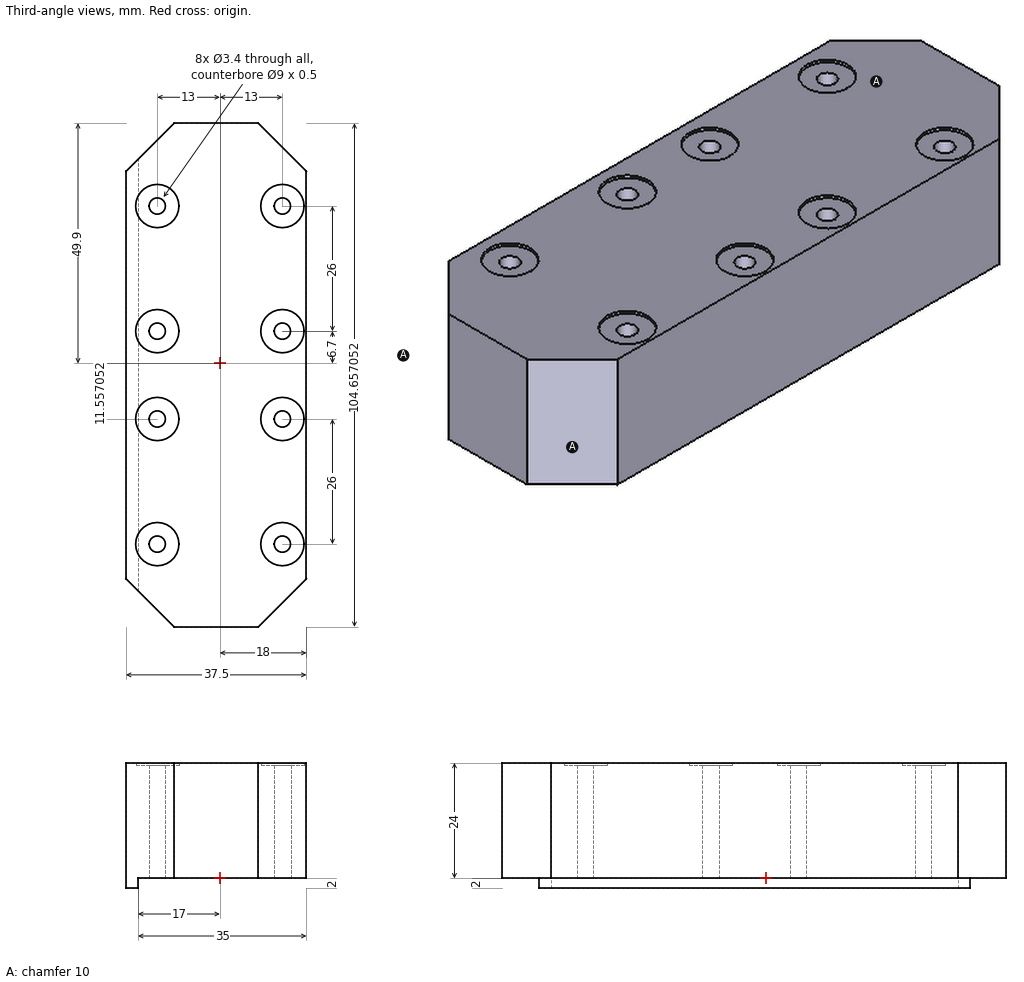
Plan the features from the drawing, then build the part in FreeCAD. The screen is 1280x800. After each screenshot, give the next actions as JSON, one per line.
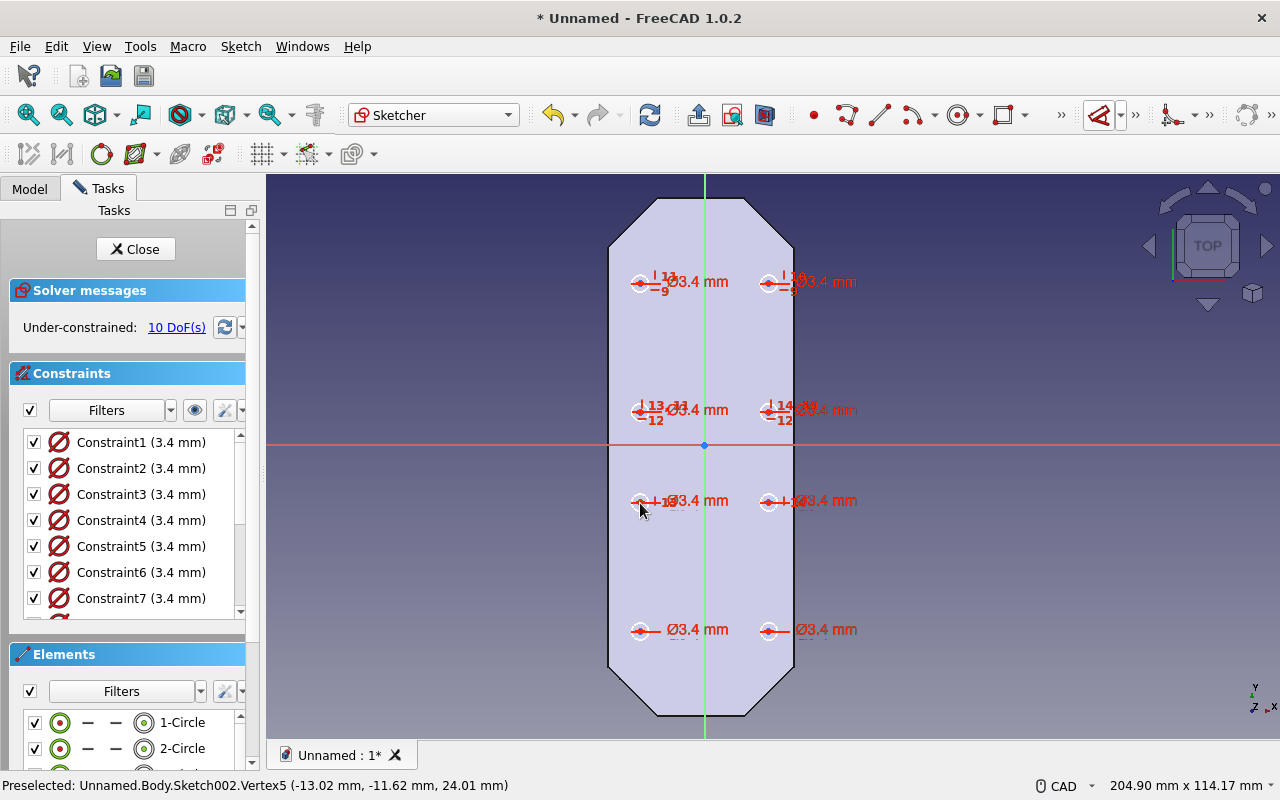
{"action": "left_click", "coordinate": [769, 503]}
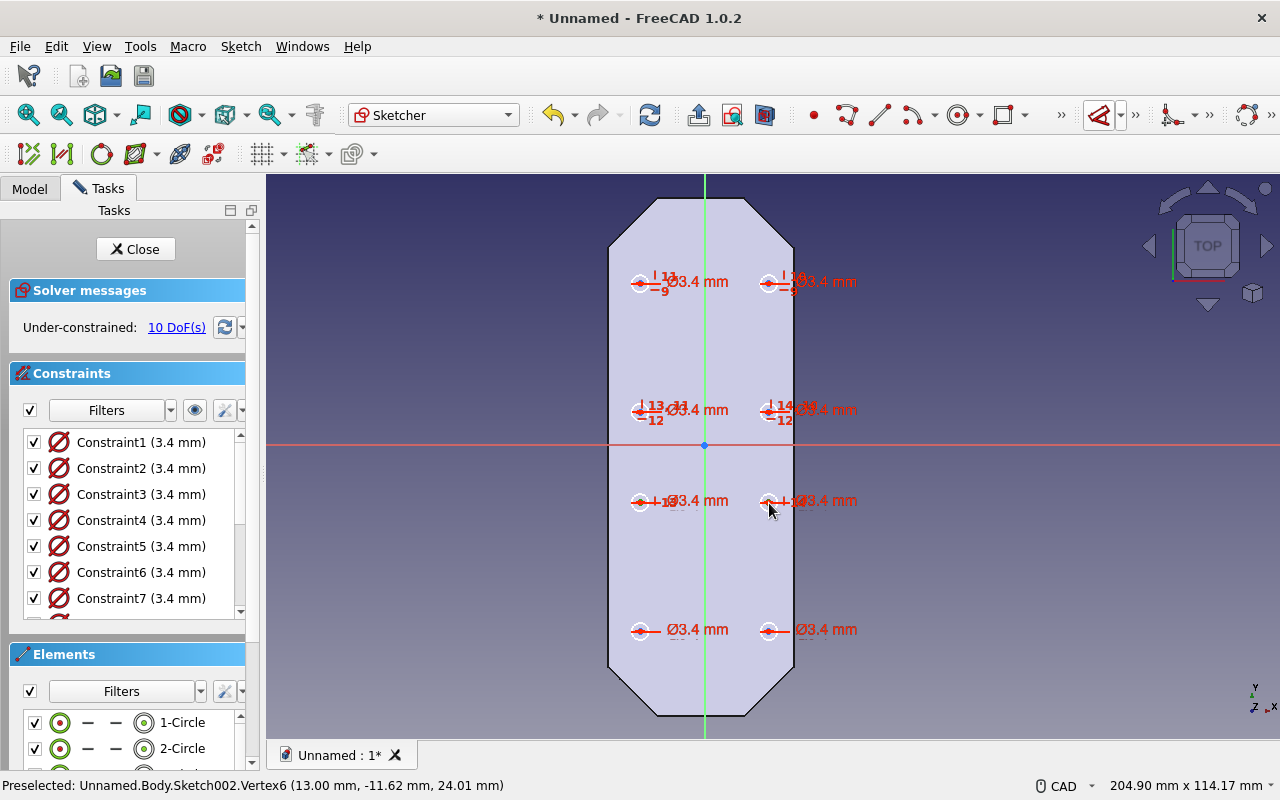
{"action": "key", "text": "h"}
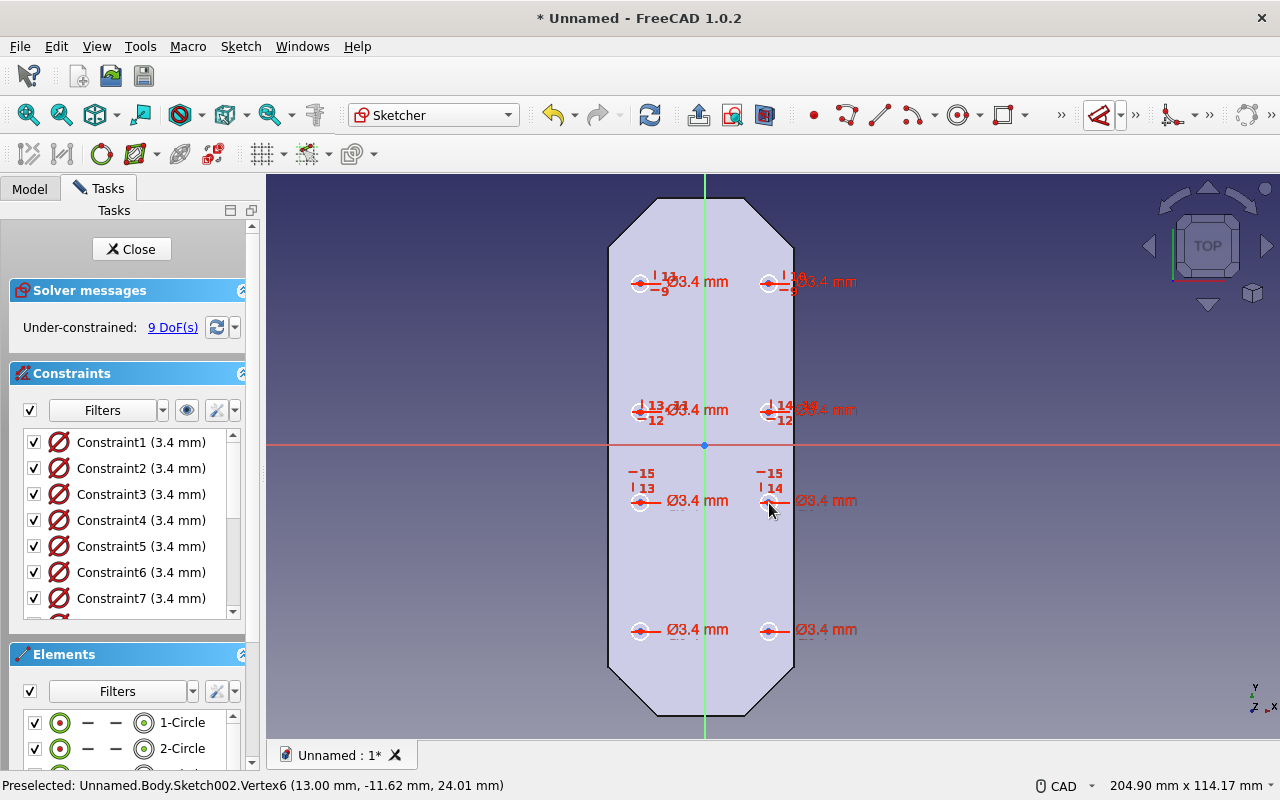
{"action": "left_click", "coordinate": [769, 503]}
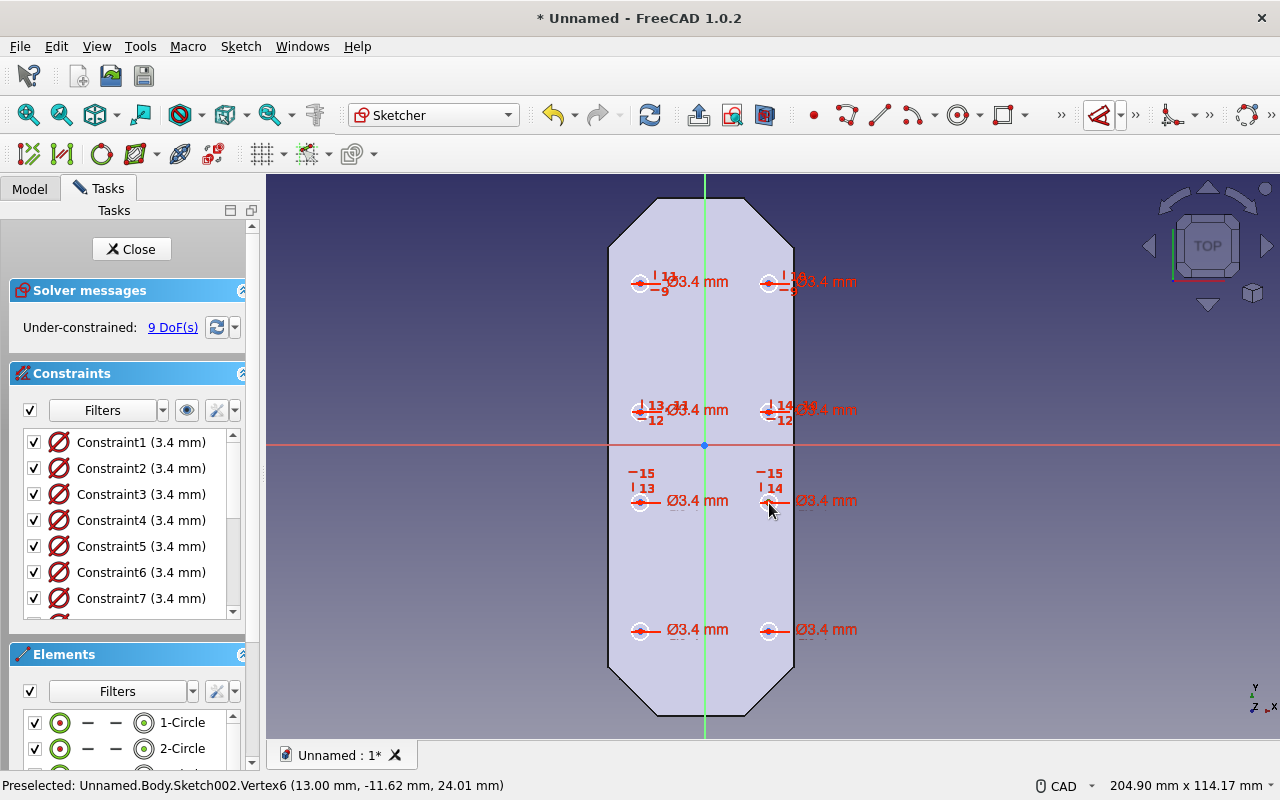
{"action": "left_click", "coordinate": [769, 632]}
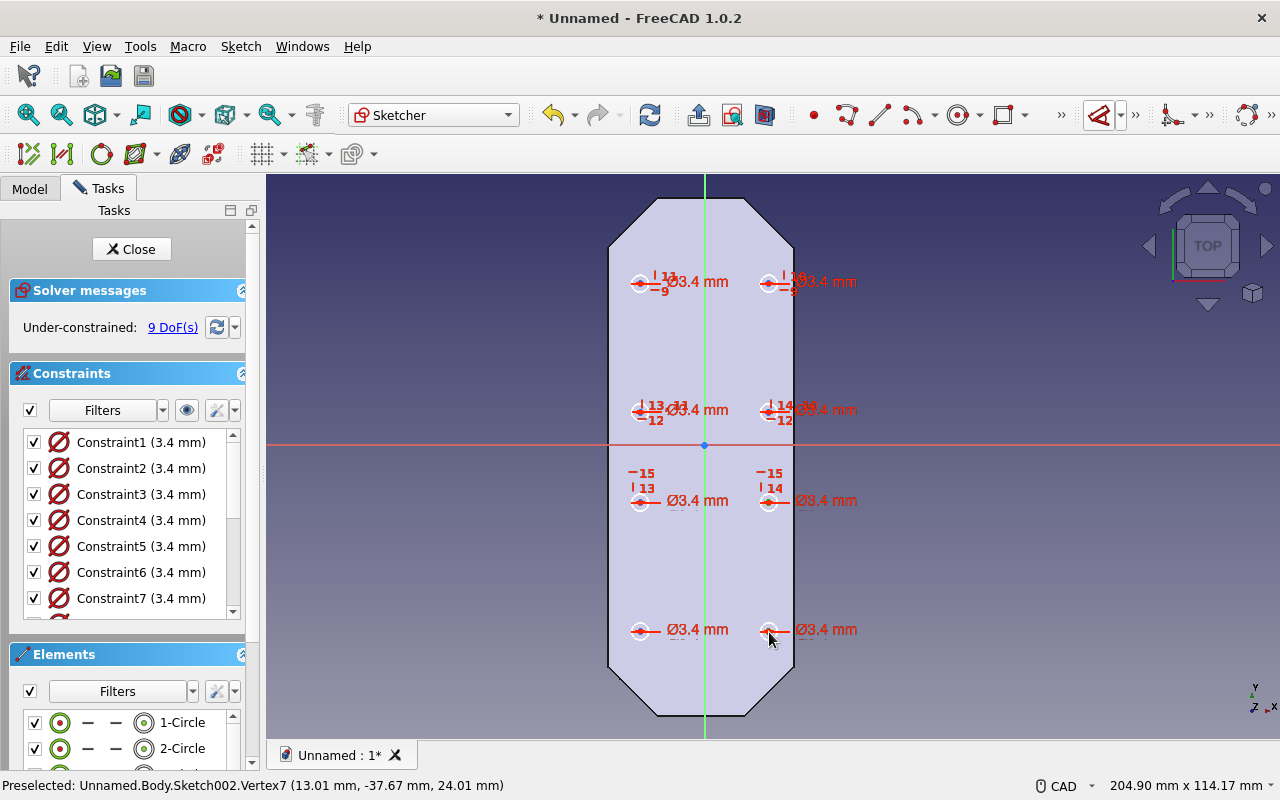
{"action": "key", "text": "v"}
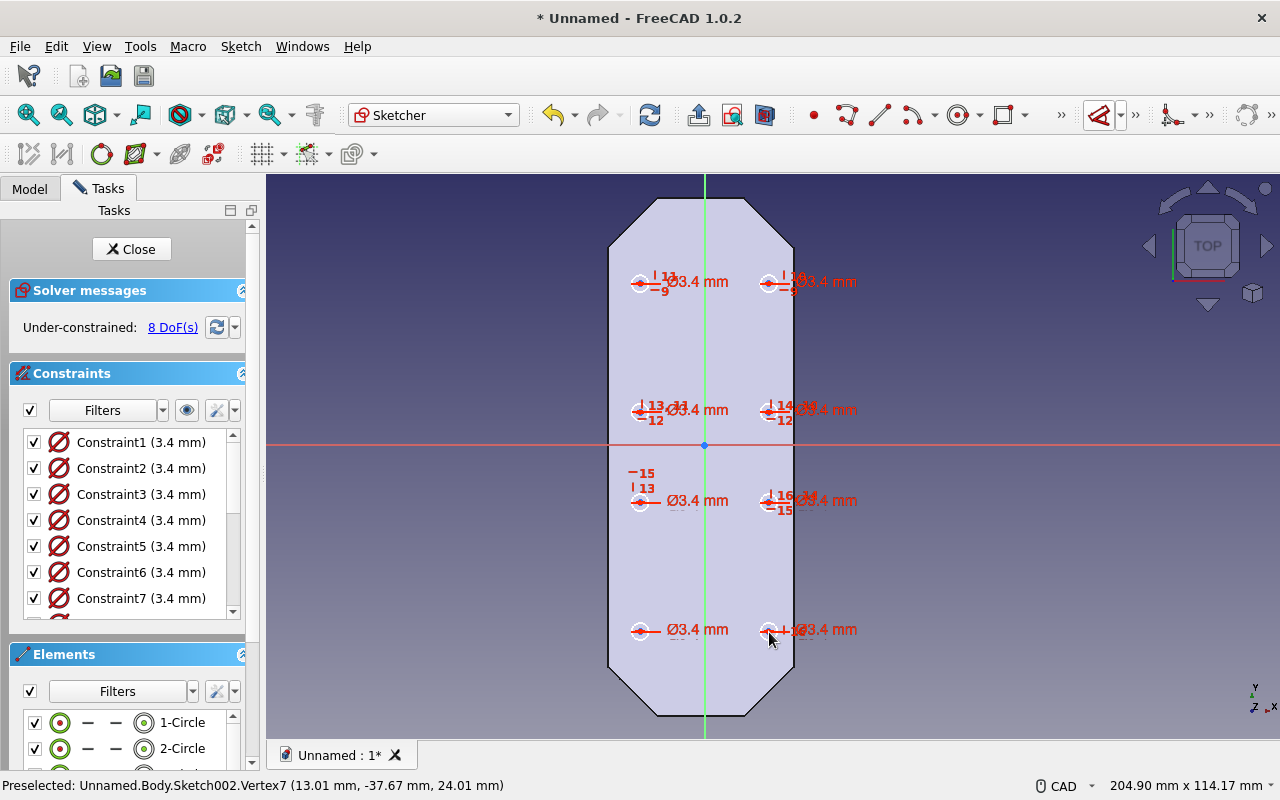
{"action": "left_click", "coordinate": [640, 503]}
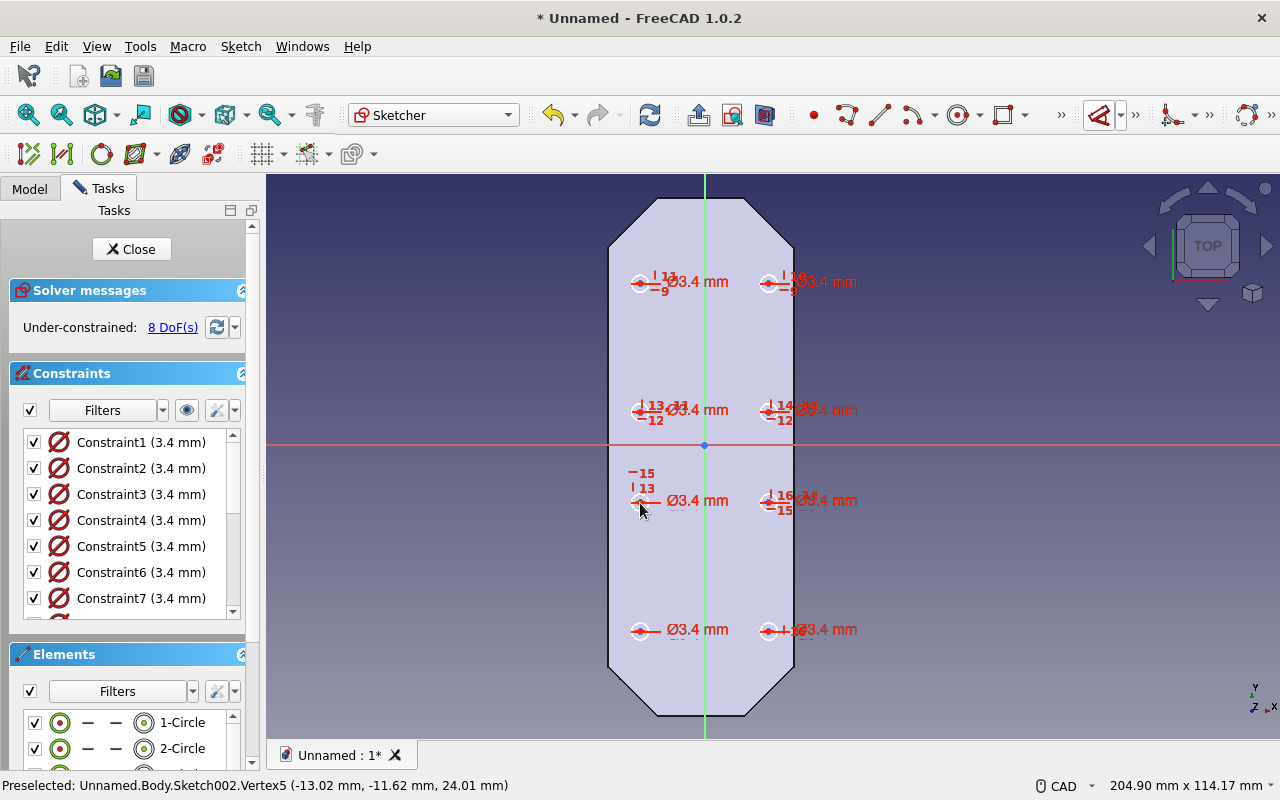
{"action": "left_click", "coordinate": [640, 632]}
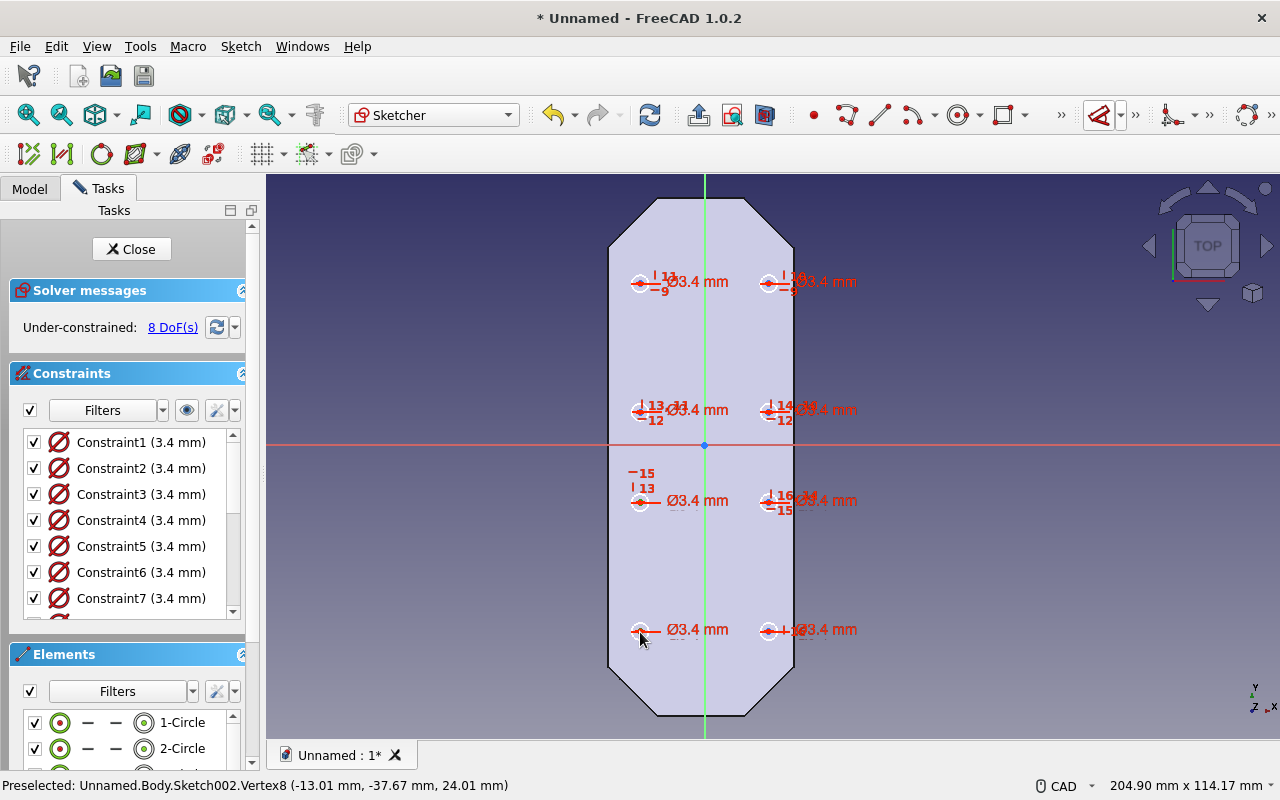
{"action": "key", "text": "v"}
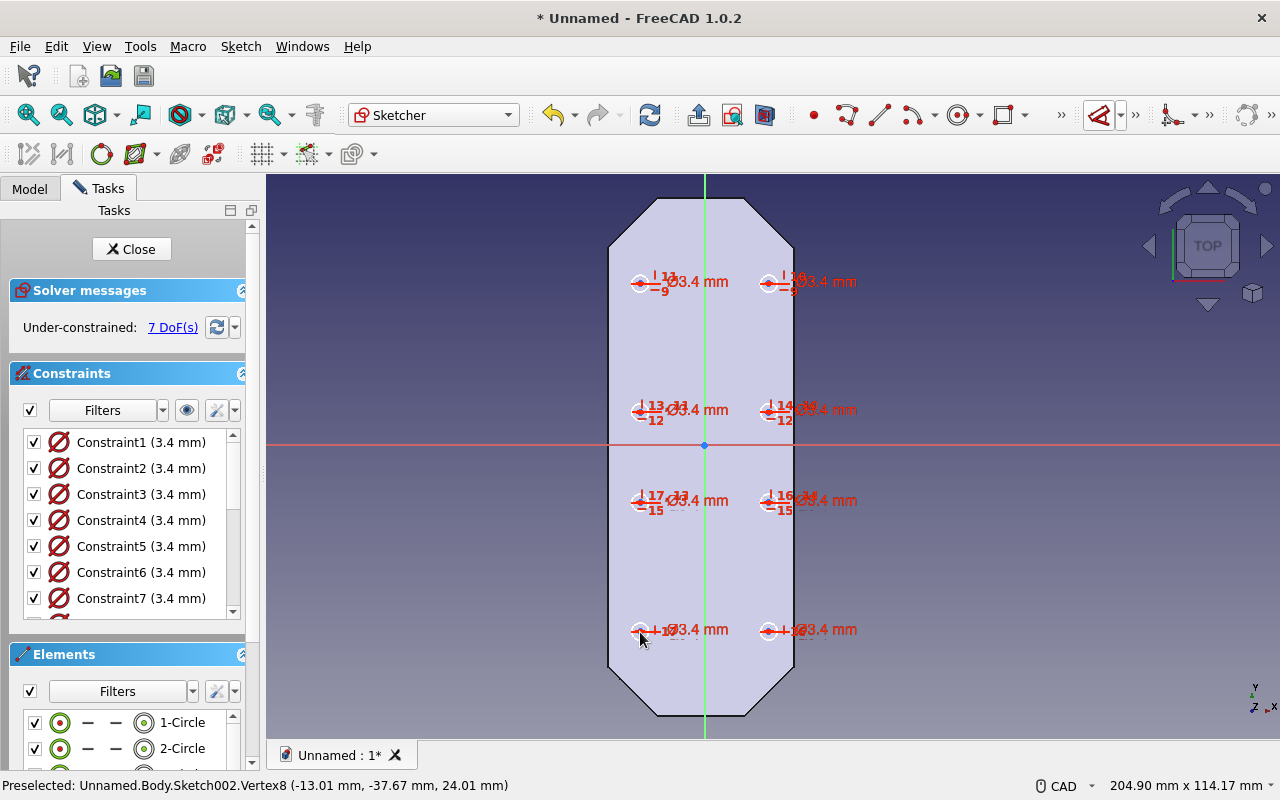
{"action": "left_click", "coordinate": [769, 632]}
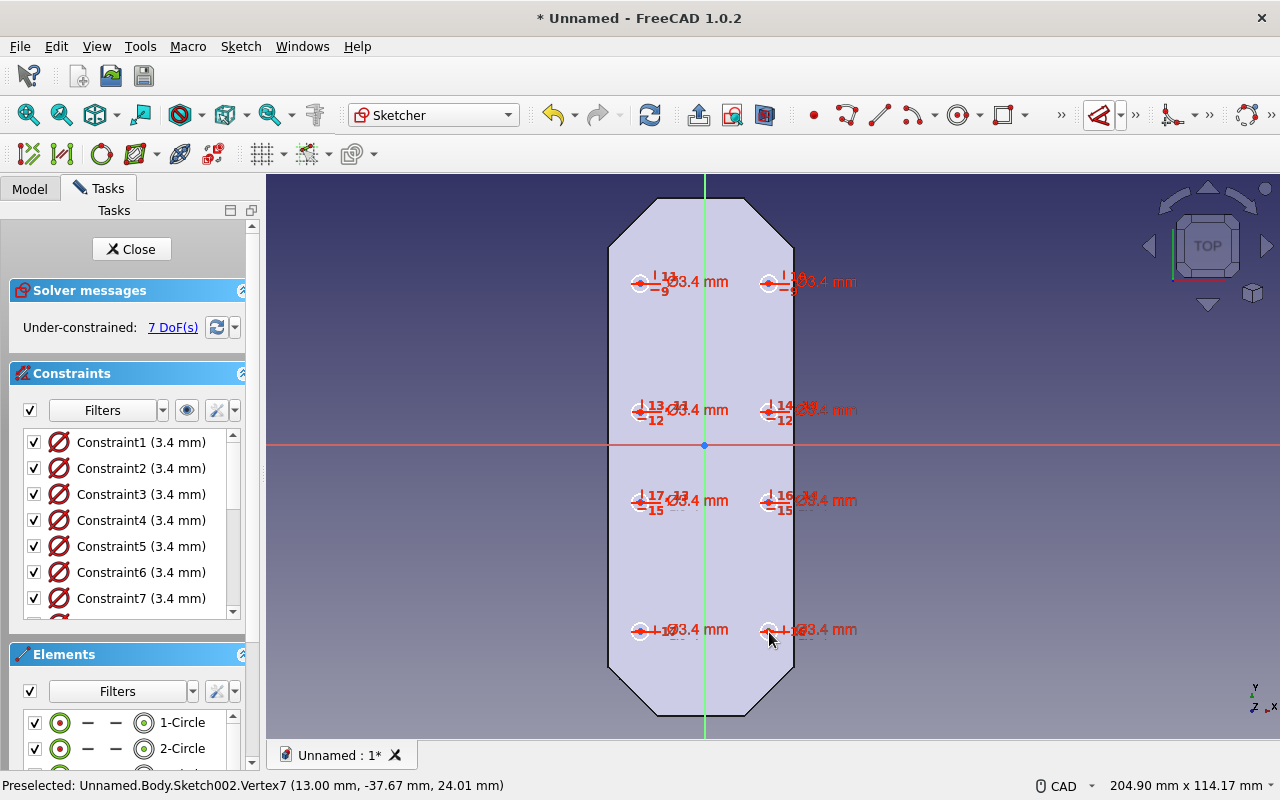
{"action": "left_click", "coordinate": [640, 632]}